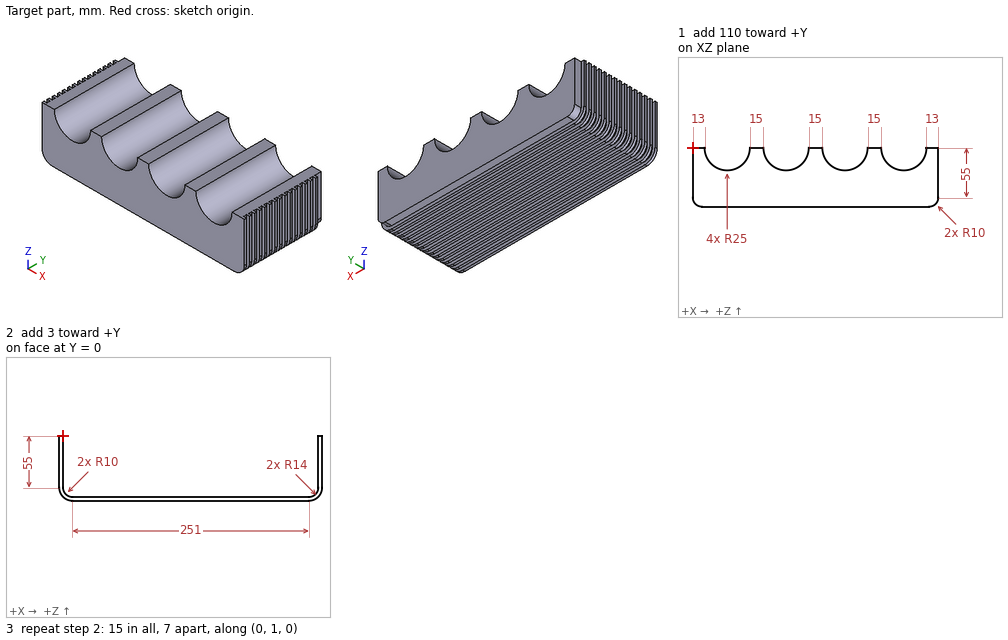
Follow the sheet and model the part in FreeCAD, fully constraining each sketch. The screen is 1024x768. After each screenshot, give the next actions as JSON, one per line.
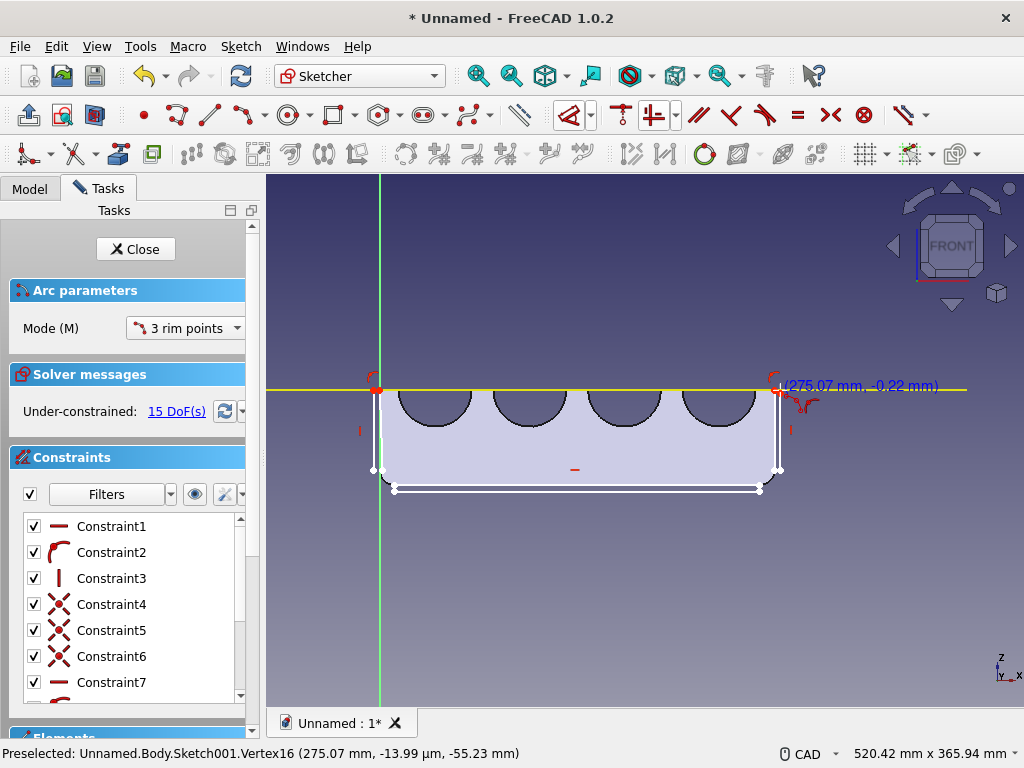
{"action": "scroll", "coordinate": [394, 491], "scroll_direction": "up", "scroll_amount": 6}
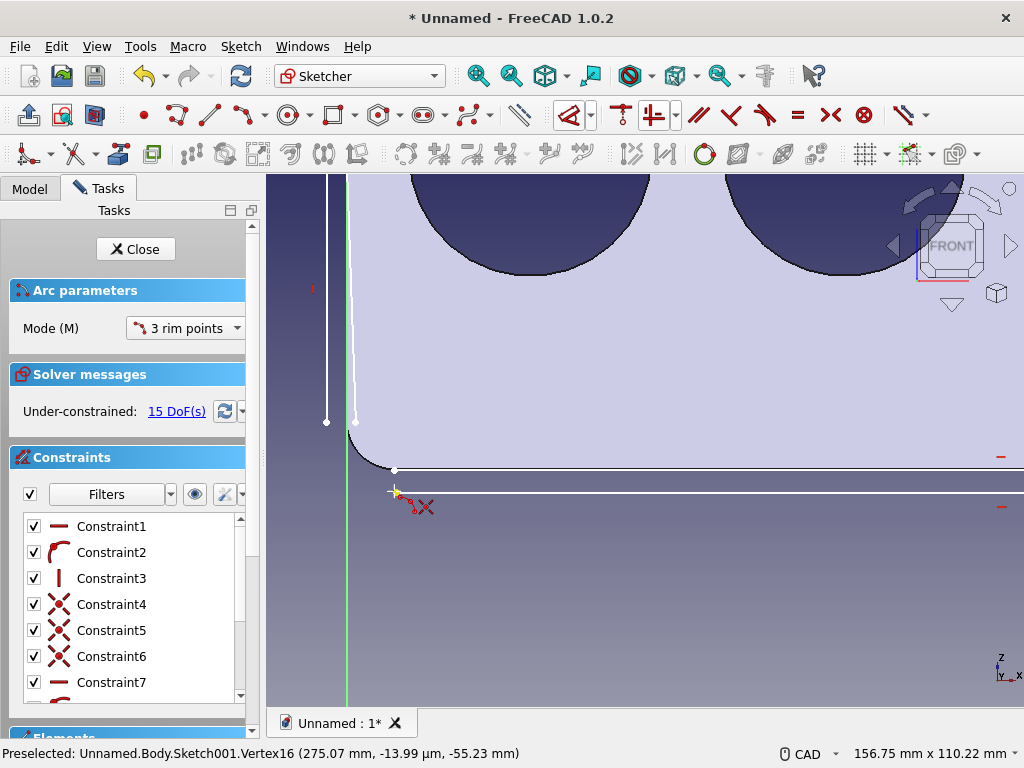
{"action": "left_click", "coordinate": [396, 493]}
{"action": "left_click", "coordinate": [327, 422]}
{"action": "left_click", "coordinate": [364, 481]}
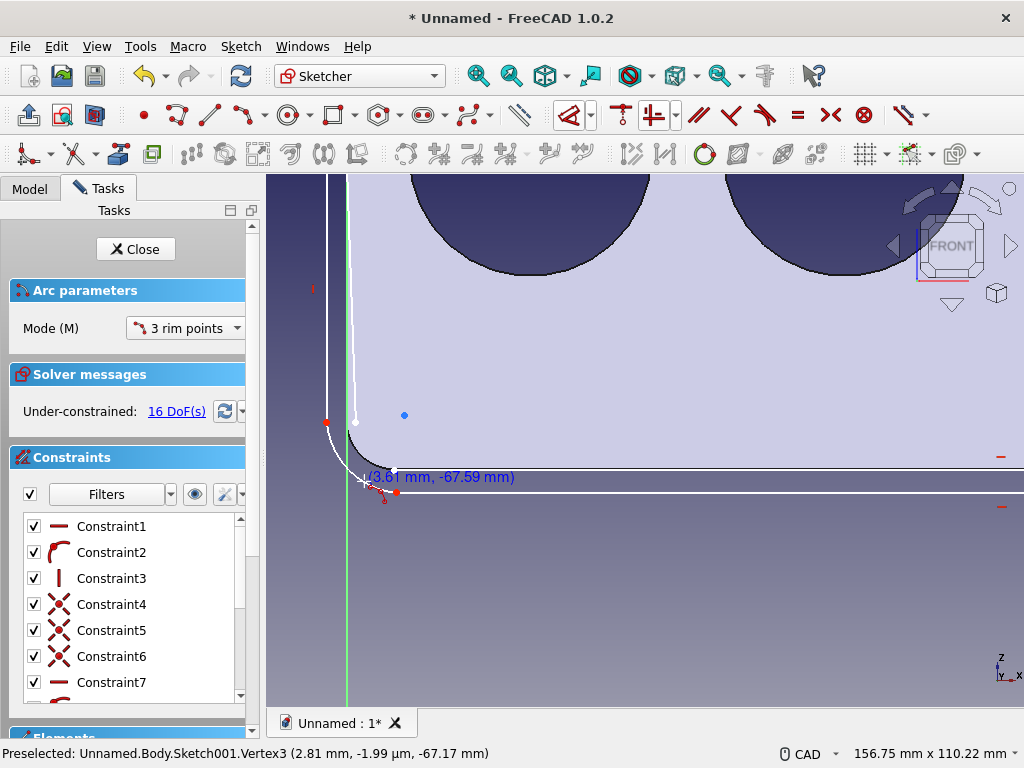
{"action": "left_click", "coordinate": [356, 422]}
{"action": "left_click", "coordinate": [395, 470]}
{"action": "left_click", "coordinate": [361, 455]}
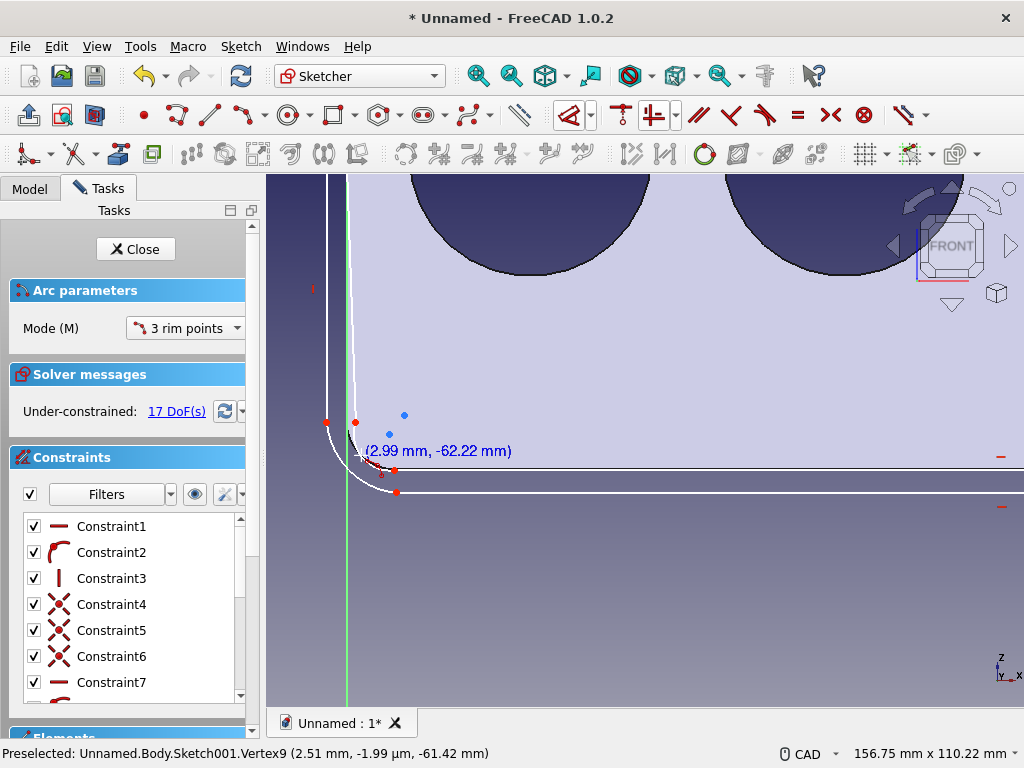
{"action": "scroll", "coordinate": [393, 492], "scroll_direction": "down", "scroll_amount": 6}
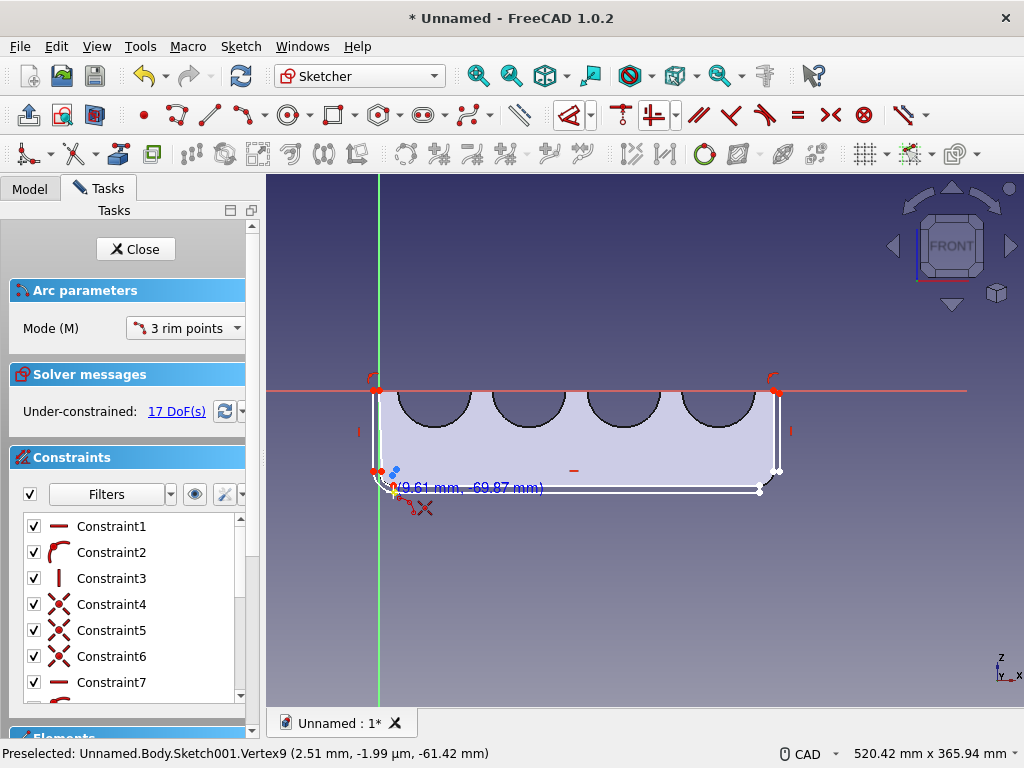
{"action": "scroll", "coordinate": [759, 486], "scroll_direction": "up", "scroll_amount": 6}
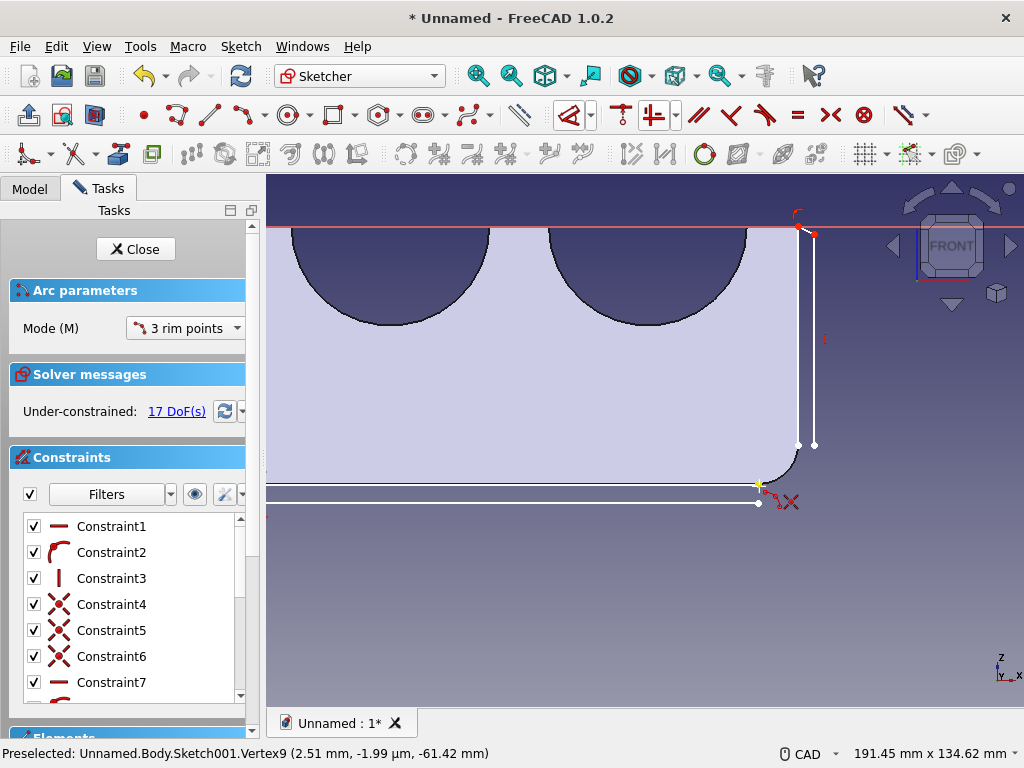
{"action": "left_click", "coordinate": [758, 484]}
{"action": "left_click", "coordinate": [807, 436]}
{"action": "left_click", "coordinate": [793, 469]}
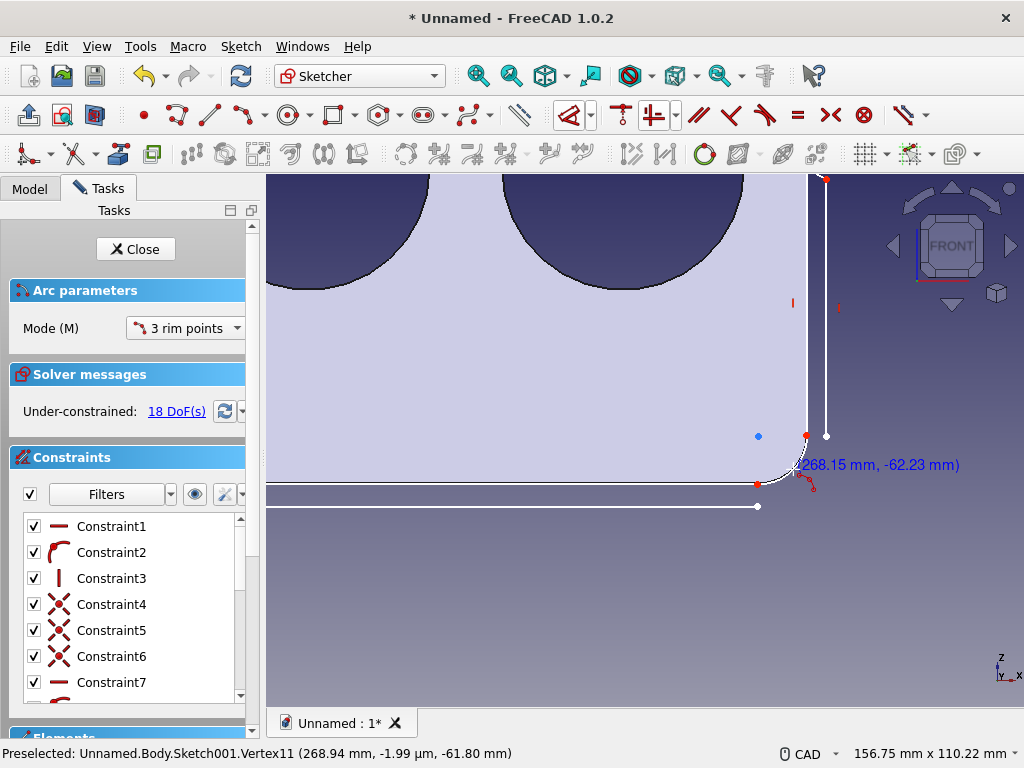
{"action": "left_click", "coordinate": [826, 436]}
{"action": "left_click", "coordinate": [758, 507]}
{"action": "left_click", "coordinate": [806, 483]}
{"action": "key", "text": "Escape"}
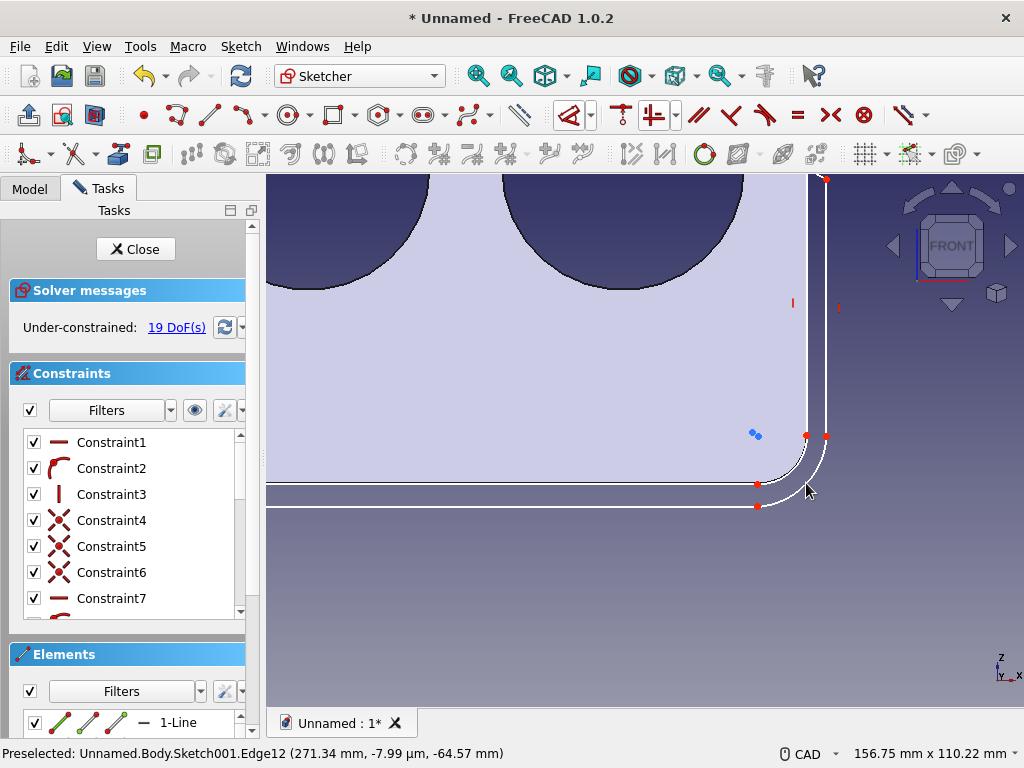
{"action": "left_click", "coordinate": [394, 507]}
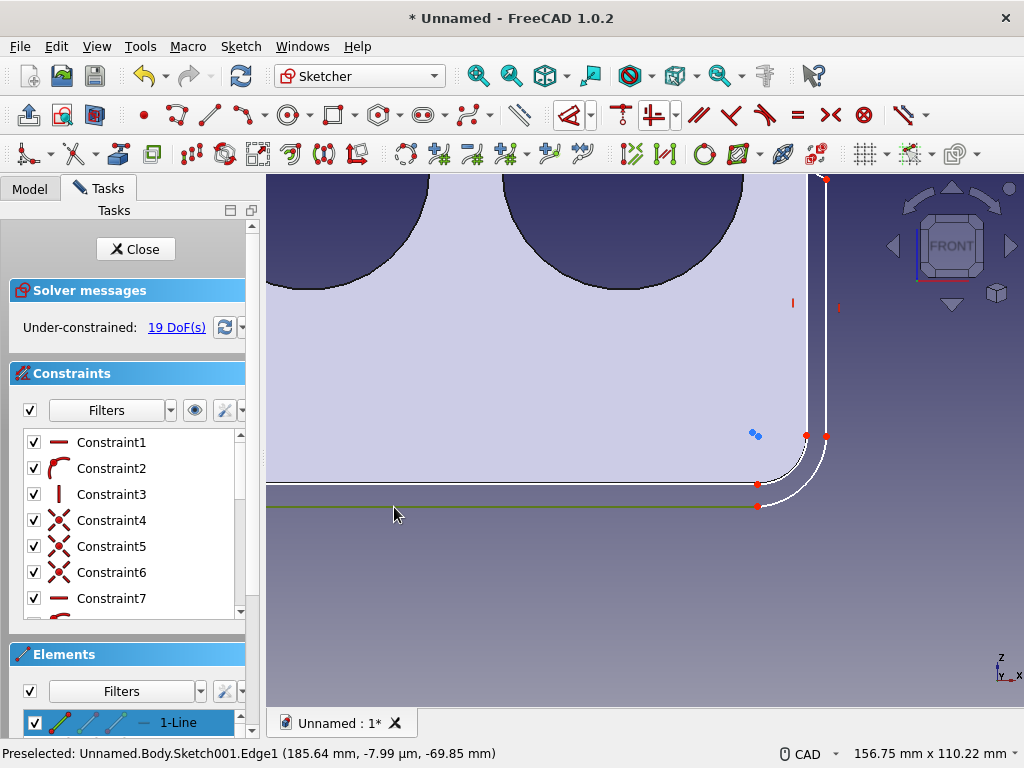
{"action": "scroll", "coordinate": [760, 486], "scroll_direction": "down", "scroll_amount": 6}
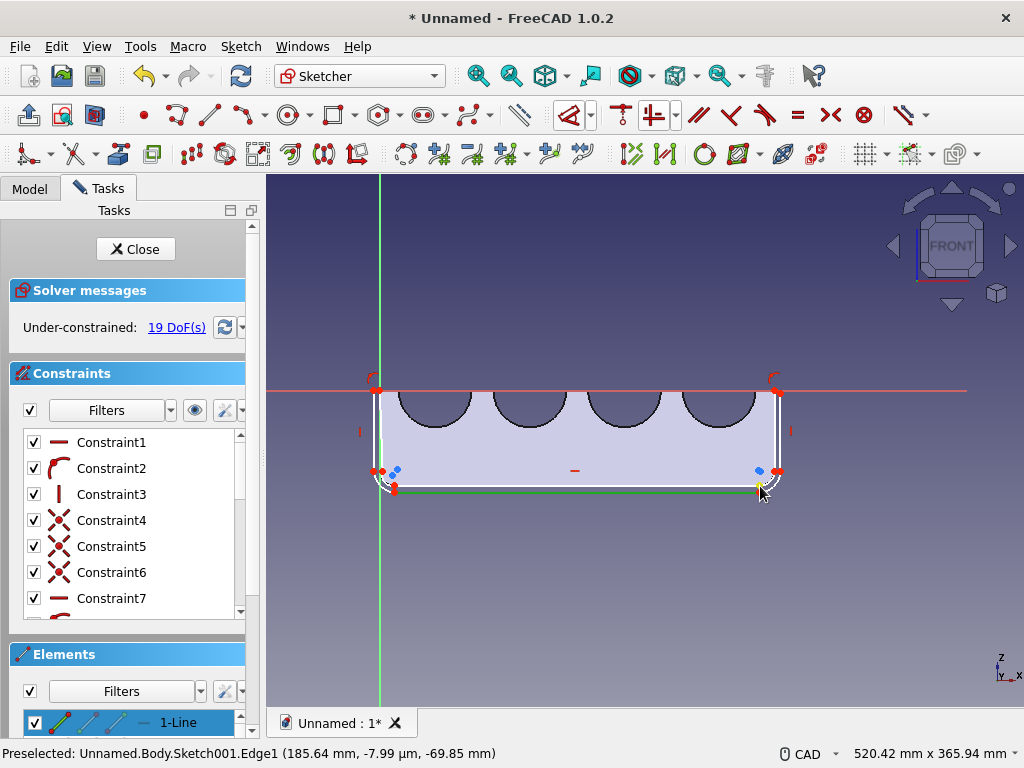
{"action": "scroll", "coordinate": [377, 481], "scroll_direction": "up", "scroll_amount": 8}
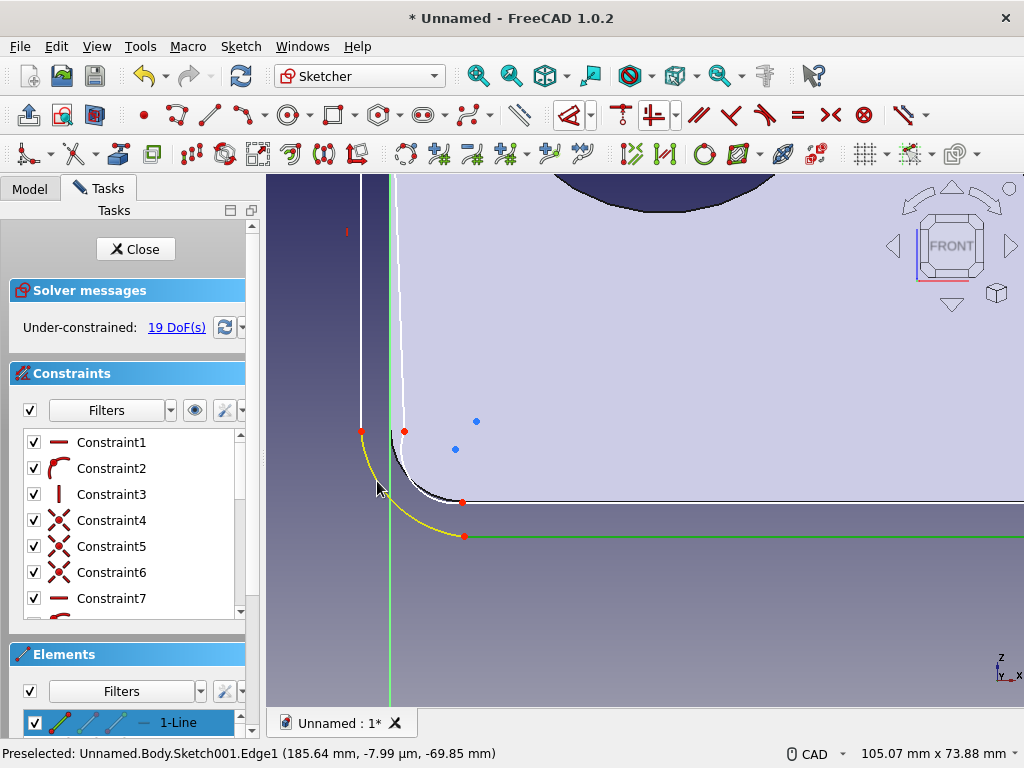
{"action": "left_click", "coordinate": [375, 477]}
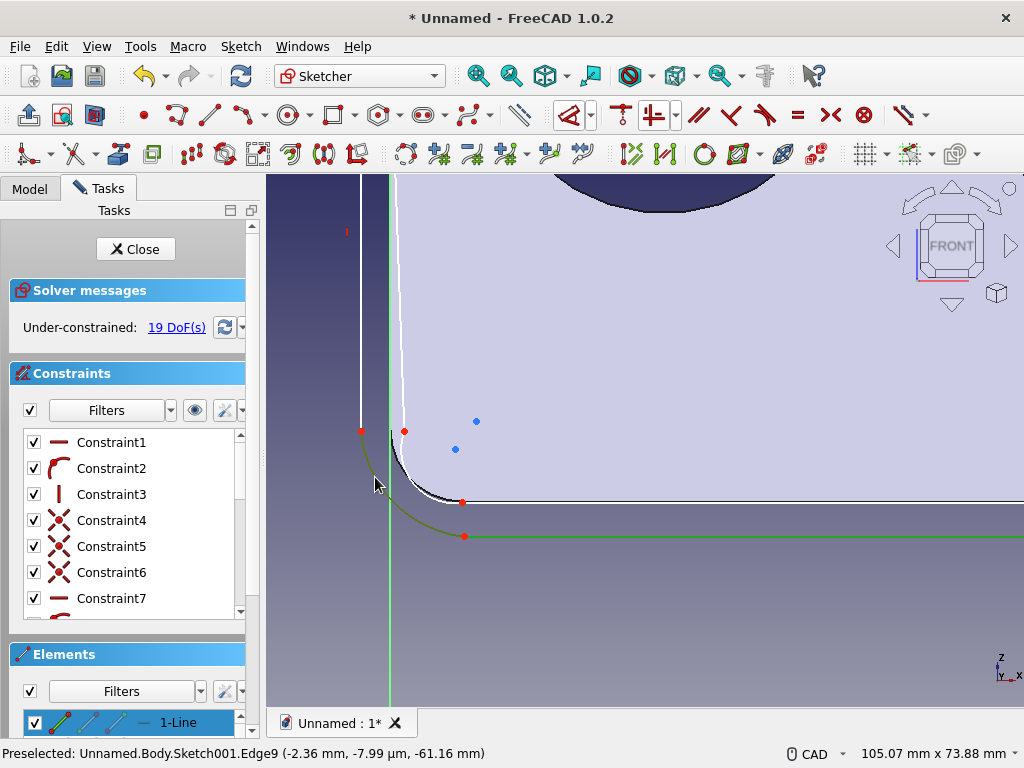
{"action": "left_click", "coordinate": [765, 116]}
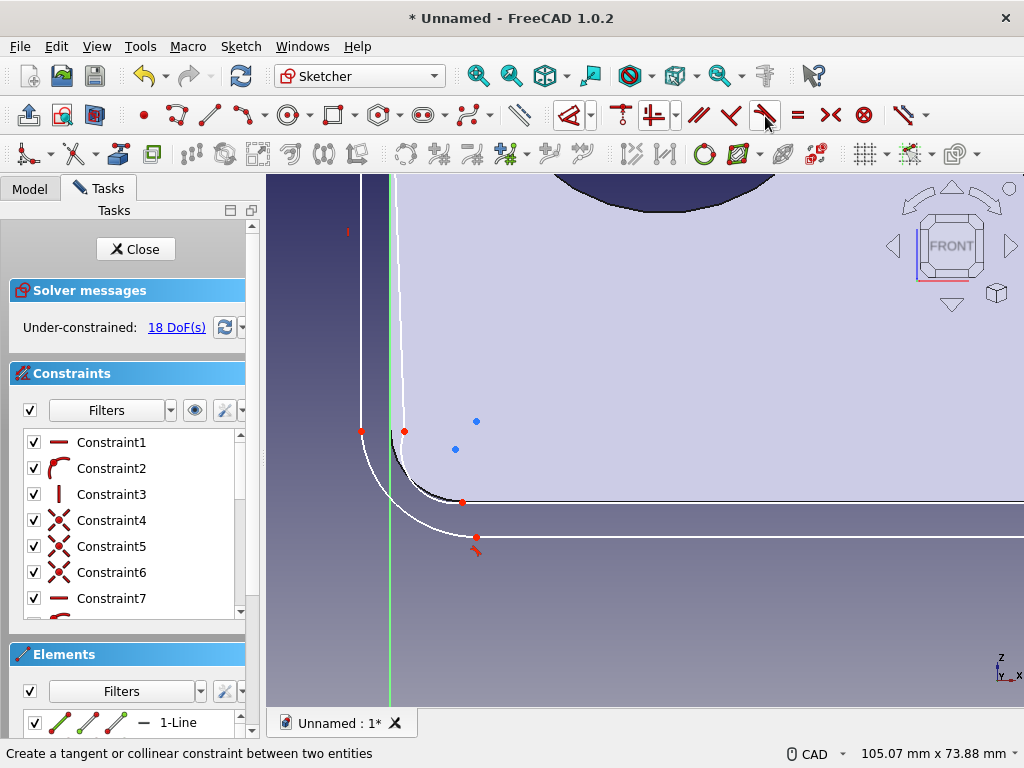
{"action": "left_click", "coordinate": [836, 537]}